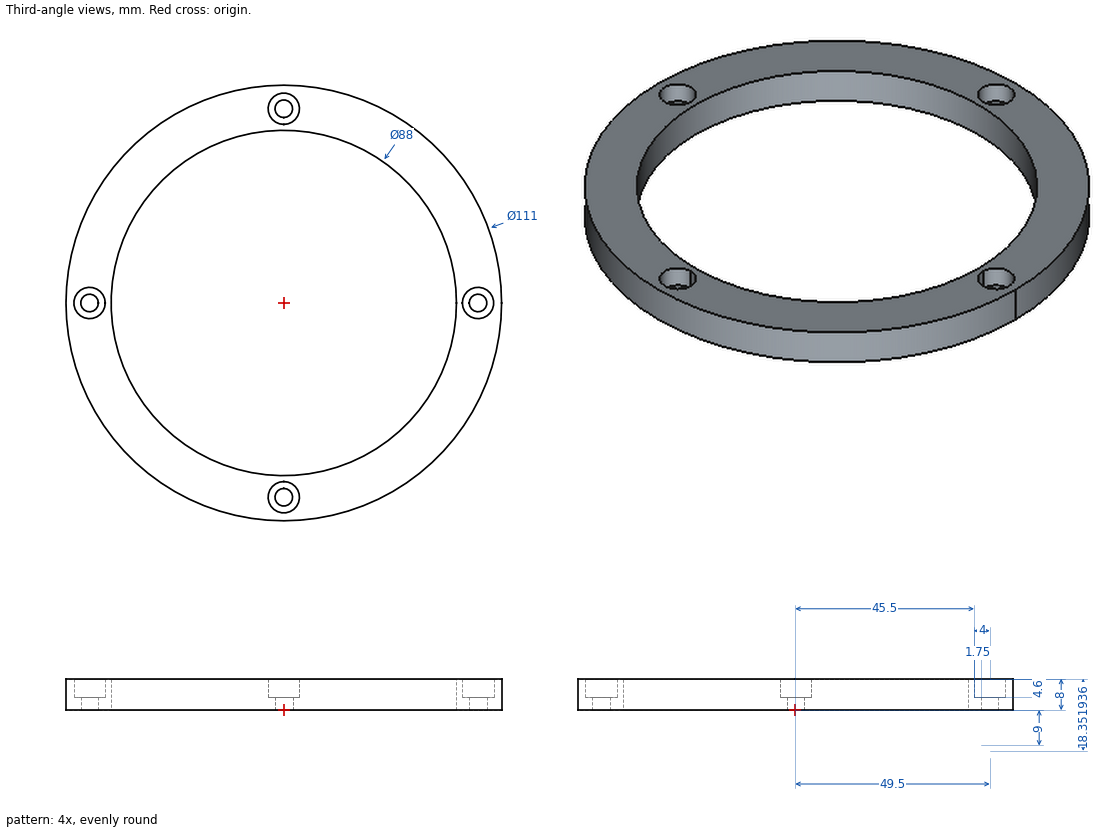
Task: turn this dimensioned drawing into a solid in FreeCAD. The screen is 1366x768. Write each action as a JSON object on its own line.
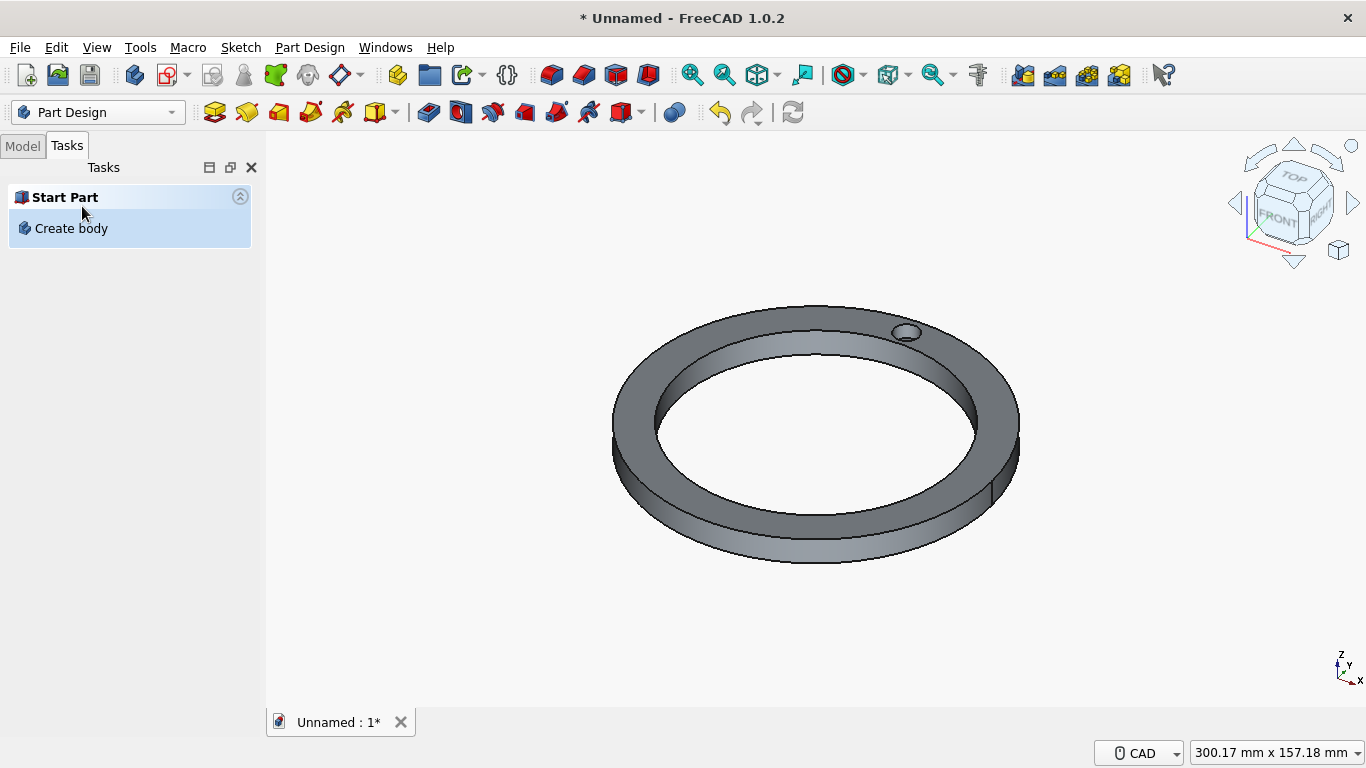
{"action": "left_click", "coordinate": [23, 145]}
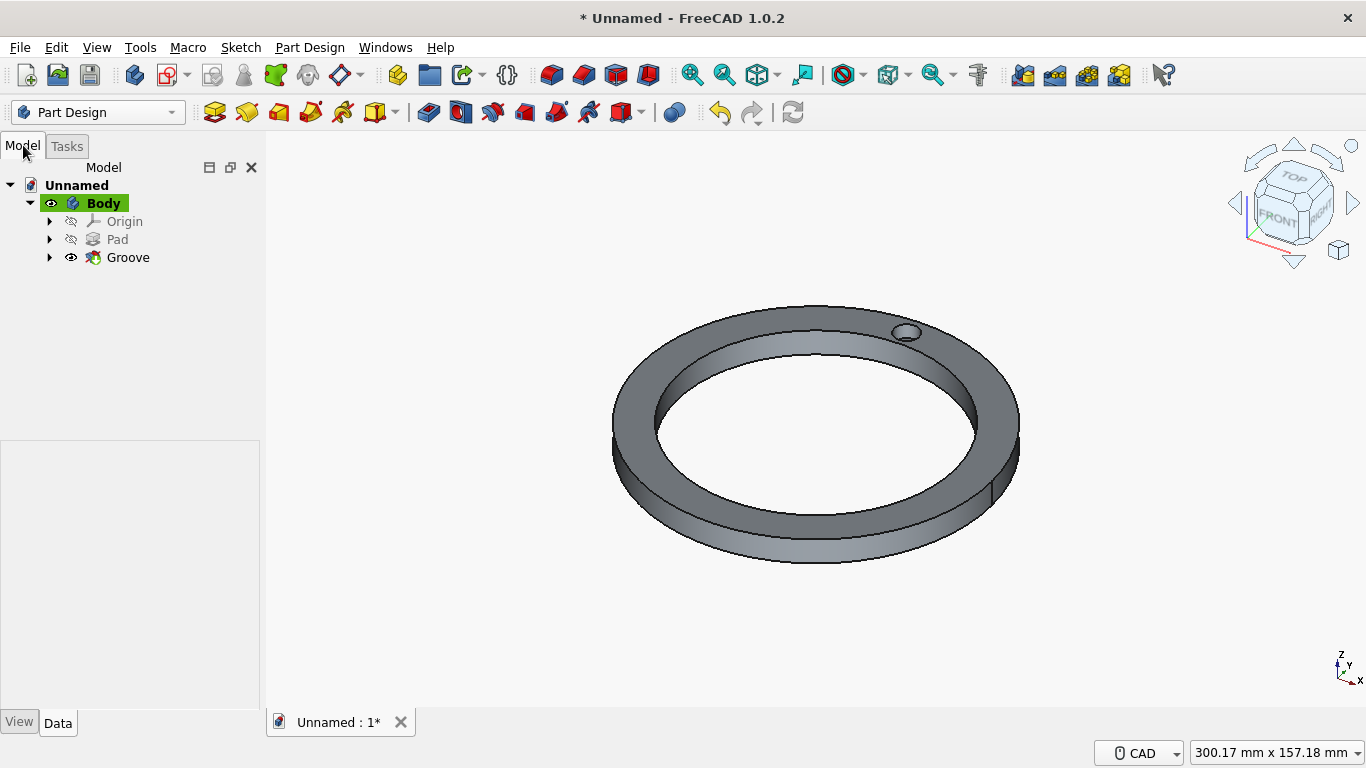
{"action": "left_click", "coordinate": [116, 257]}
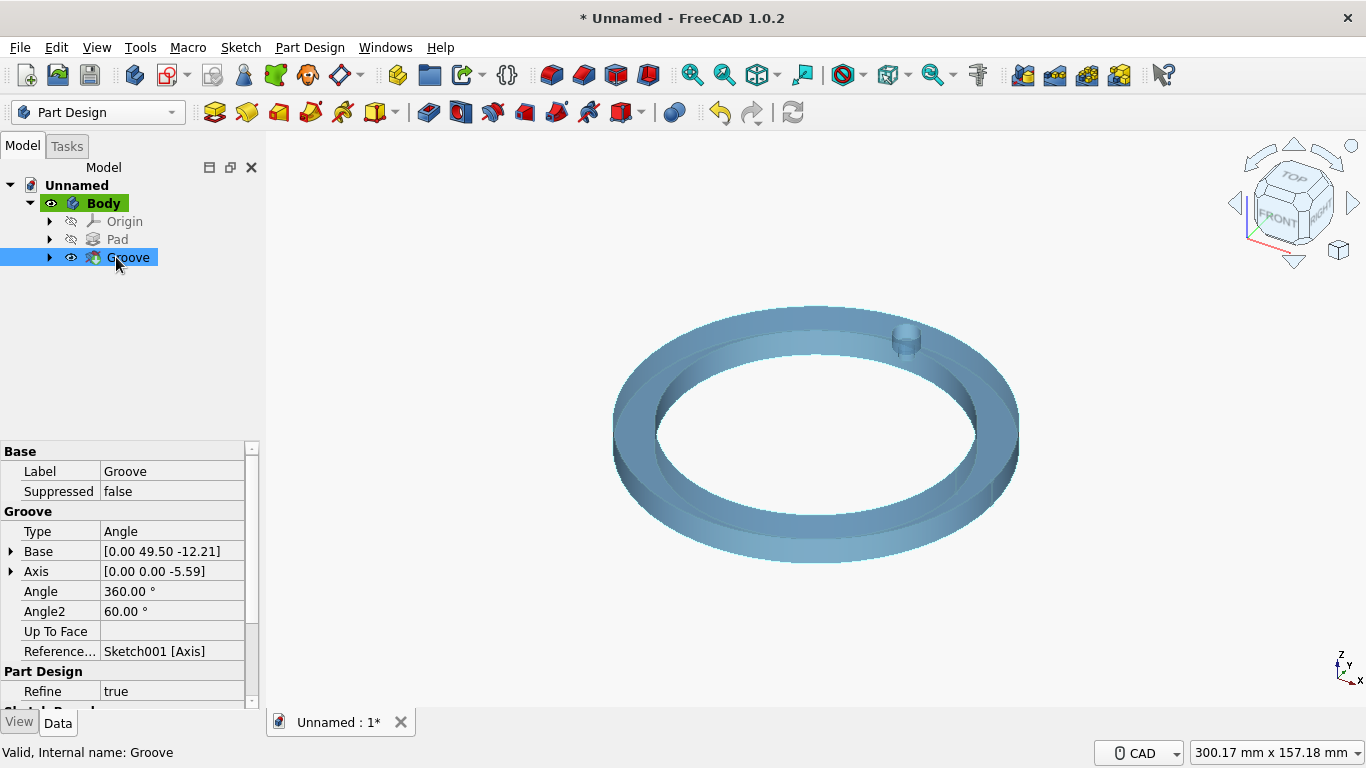
{"action": "left_click", "coordinate": [1088, 76]}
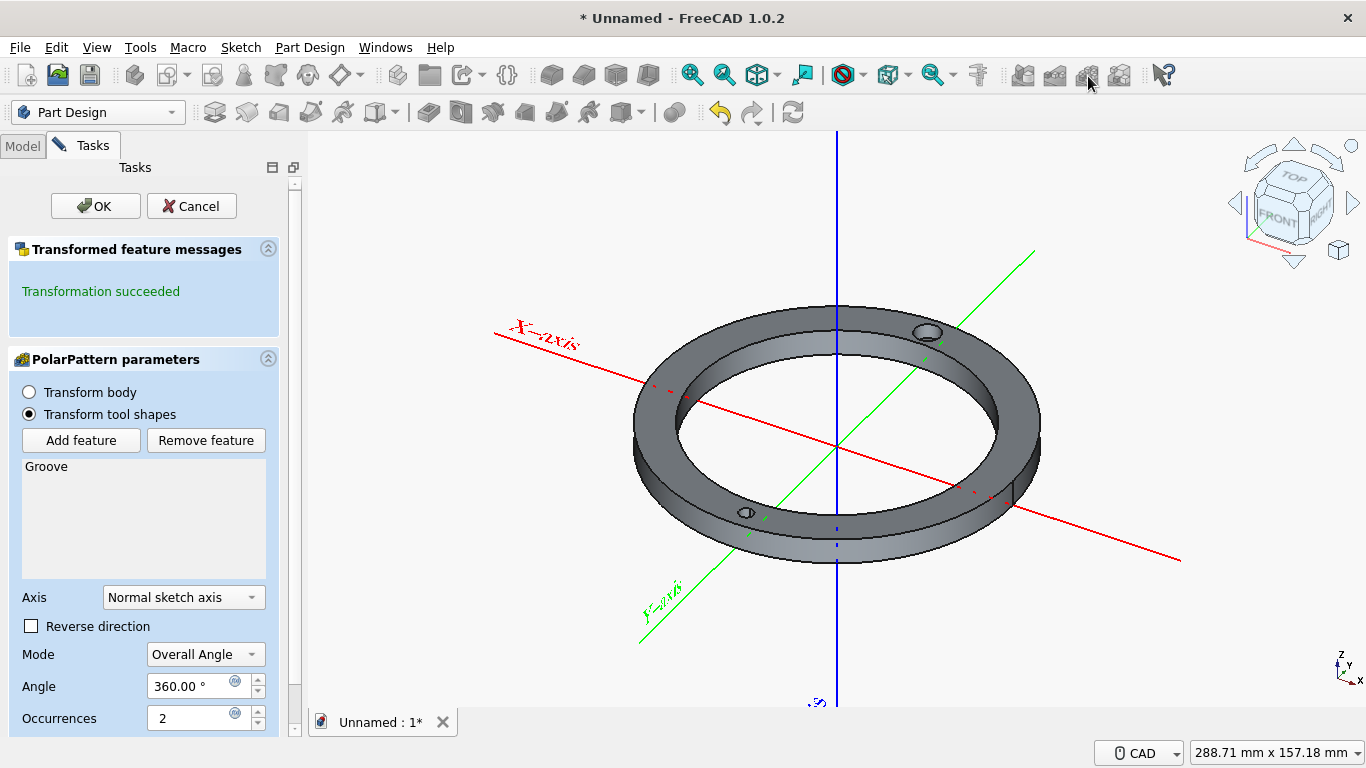
{"action": "left_click", "coordinate": [184, 598]}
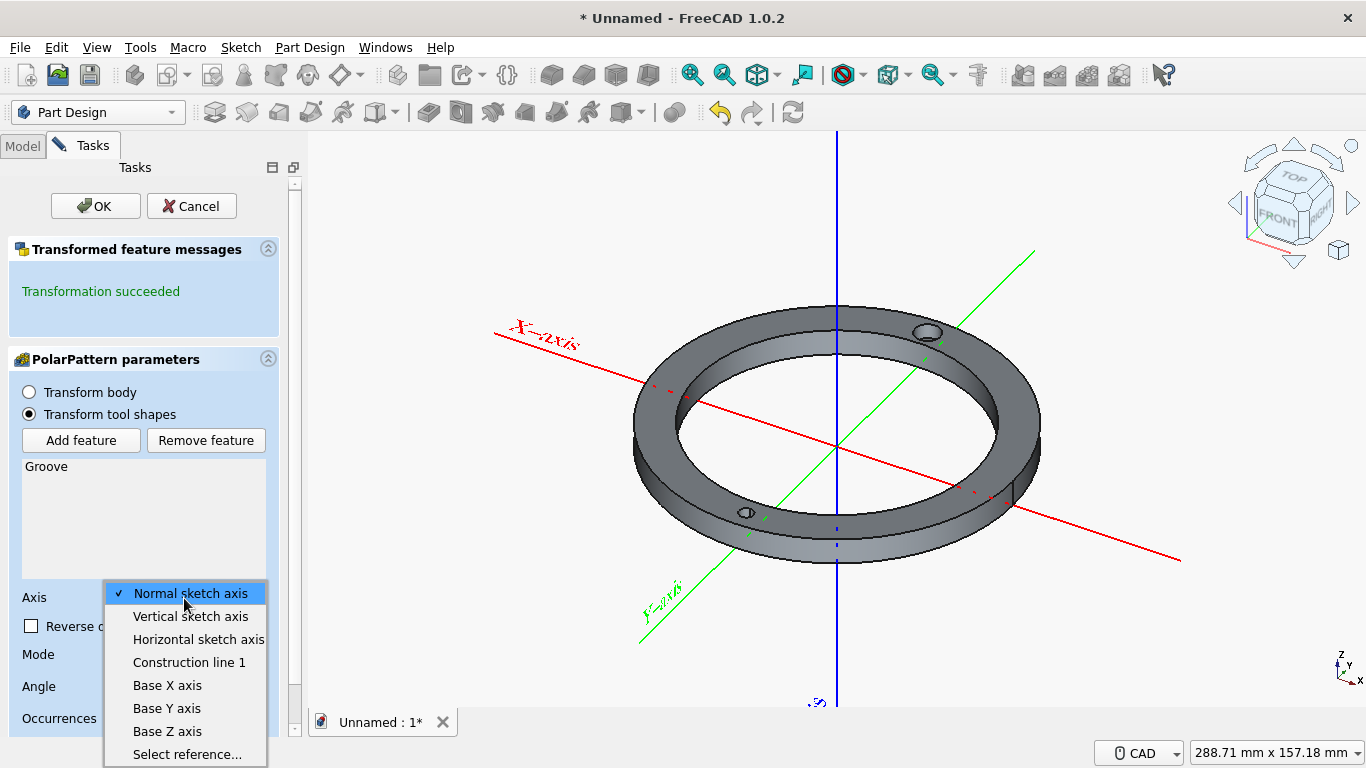
{"action": "left_click", "coordinate": [184, 732]}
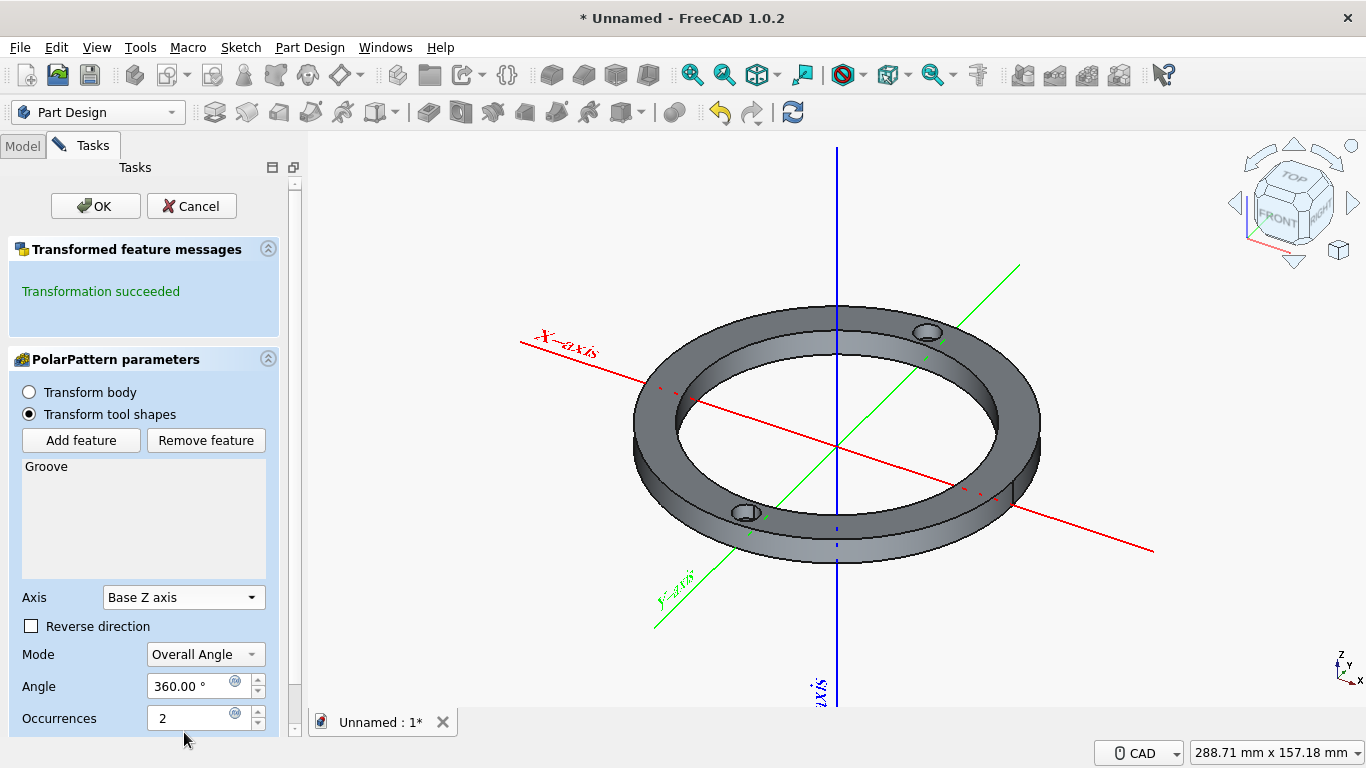
{"action": "triple_click", "coordinate": [198, 718]}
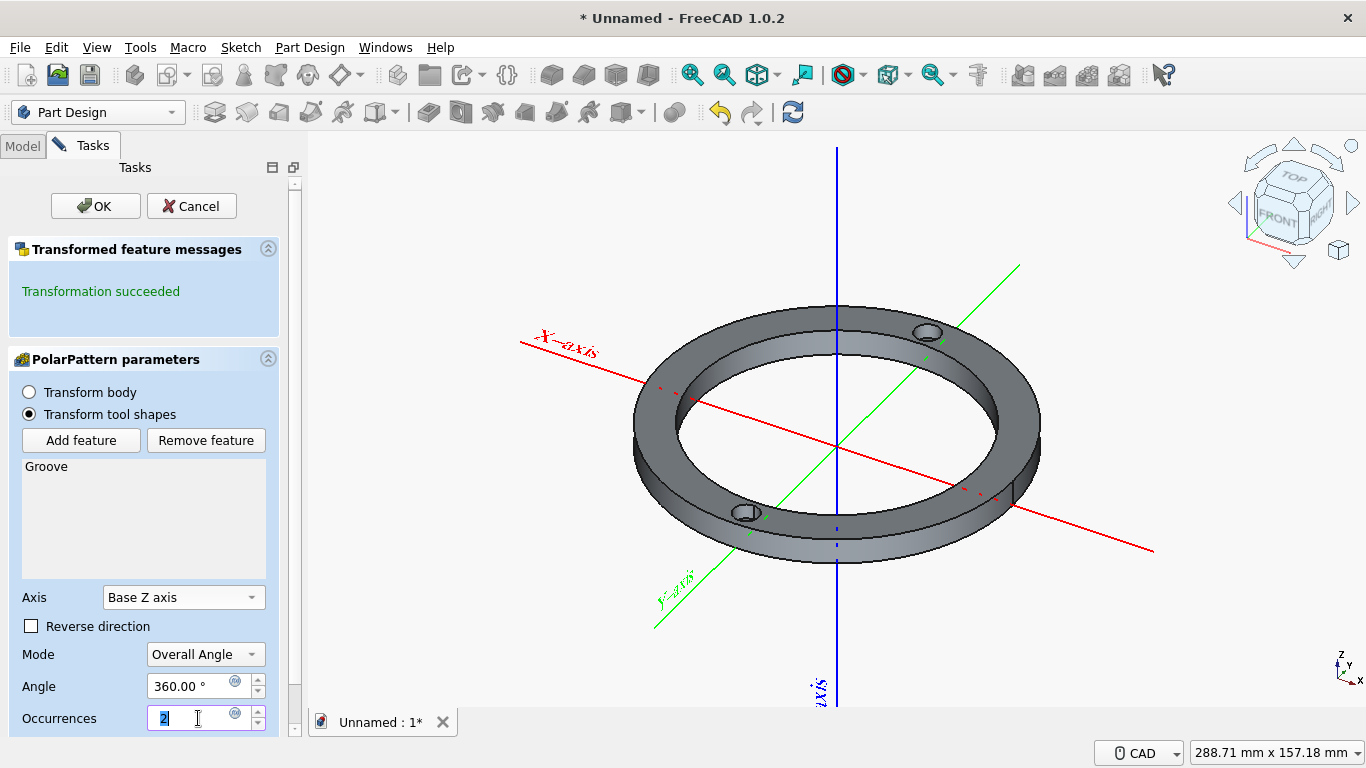
{"action": "type", "text": "4"}
{"action": "key", "text": "Tab"}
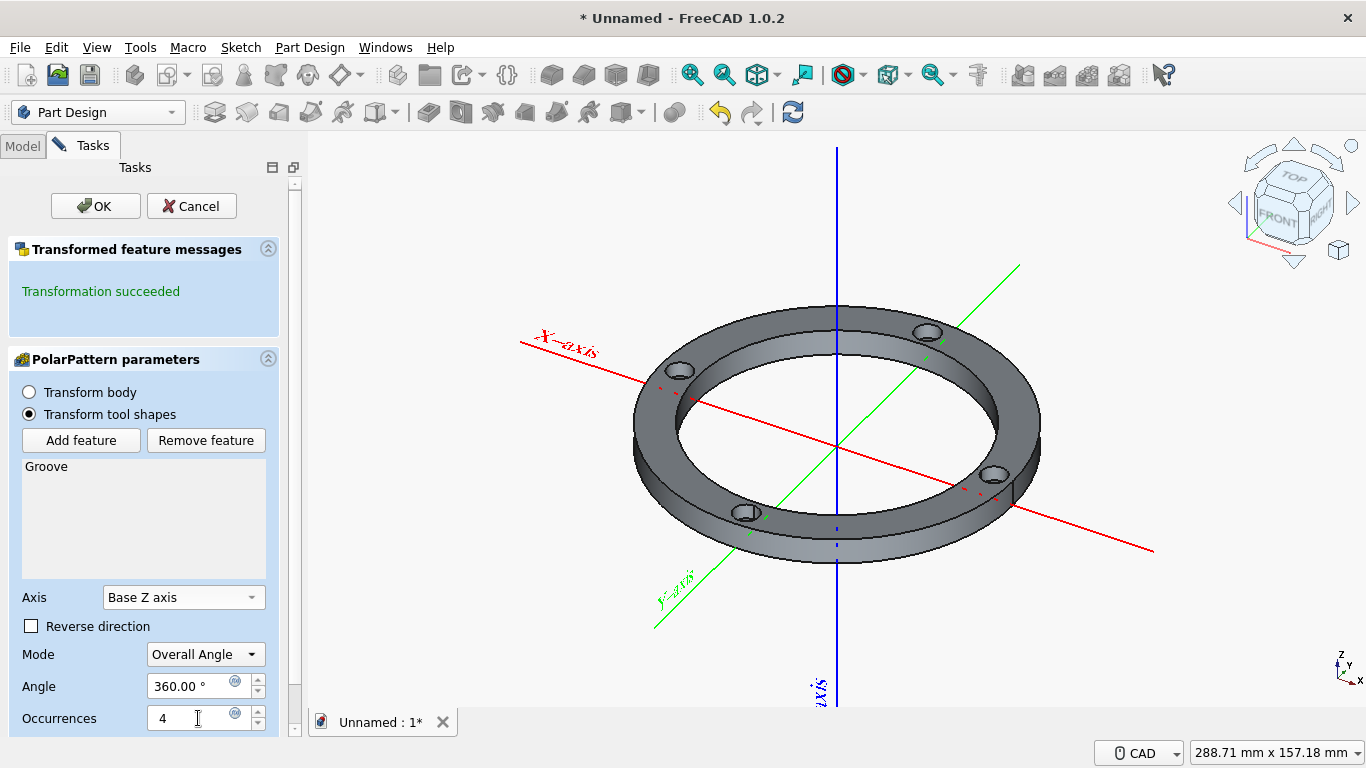
{"action": "left_click", "coordinate": [96, 206]}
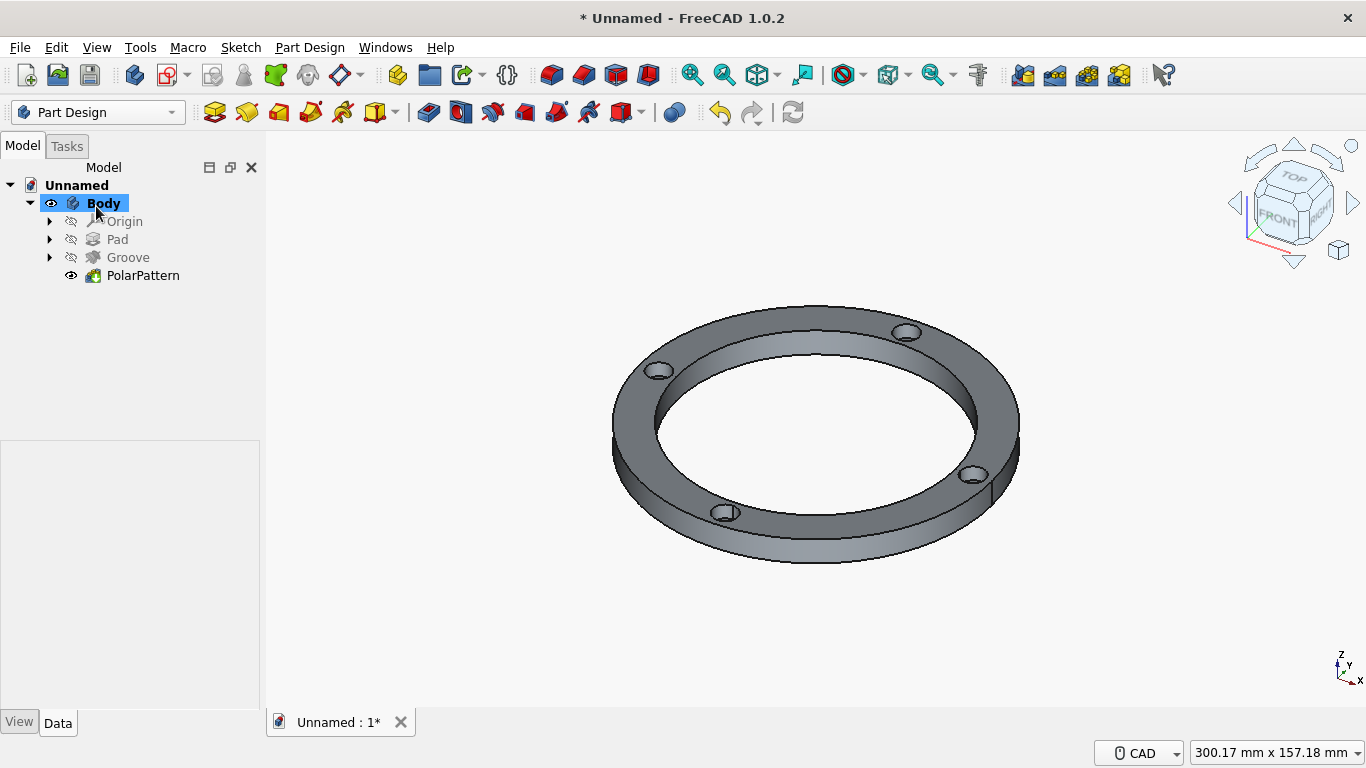
{"action": "key", "text": "0"}